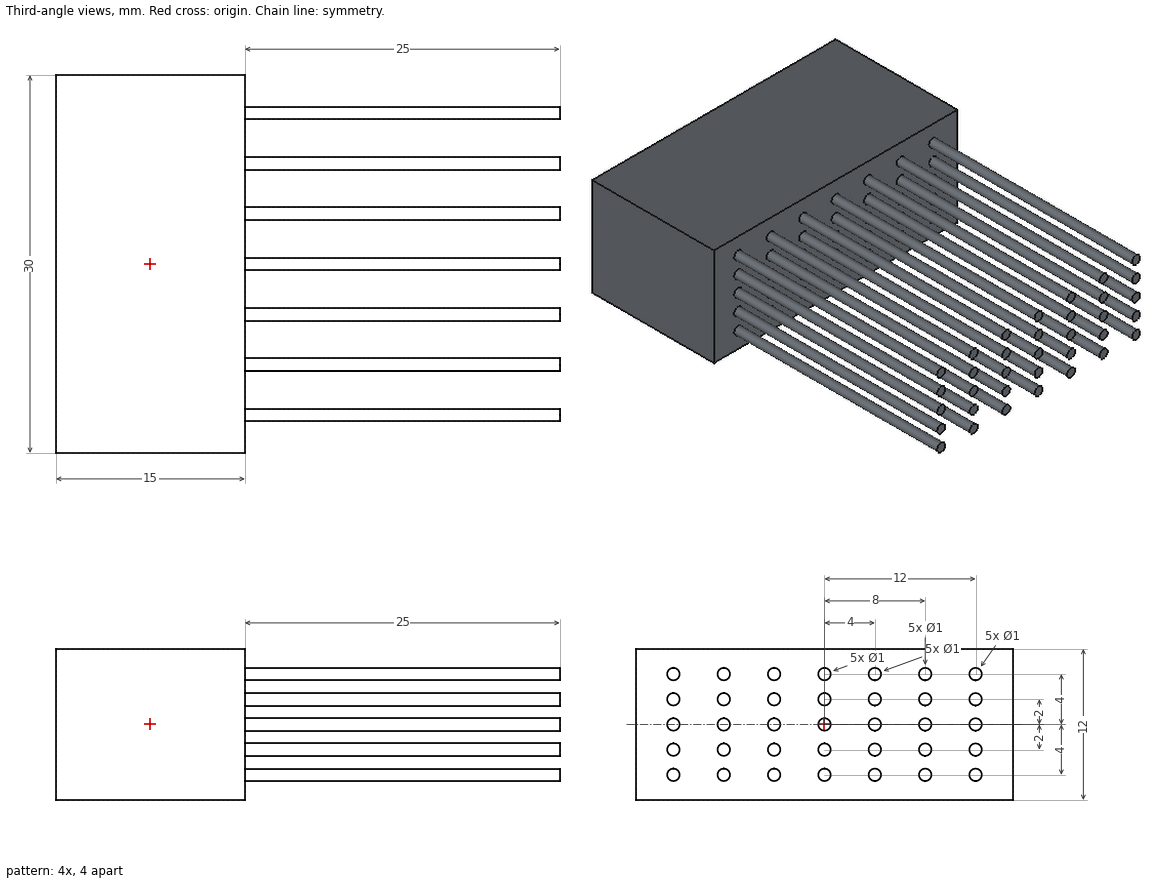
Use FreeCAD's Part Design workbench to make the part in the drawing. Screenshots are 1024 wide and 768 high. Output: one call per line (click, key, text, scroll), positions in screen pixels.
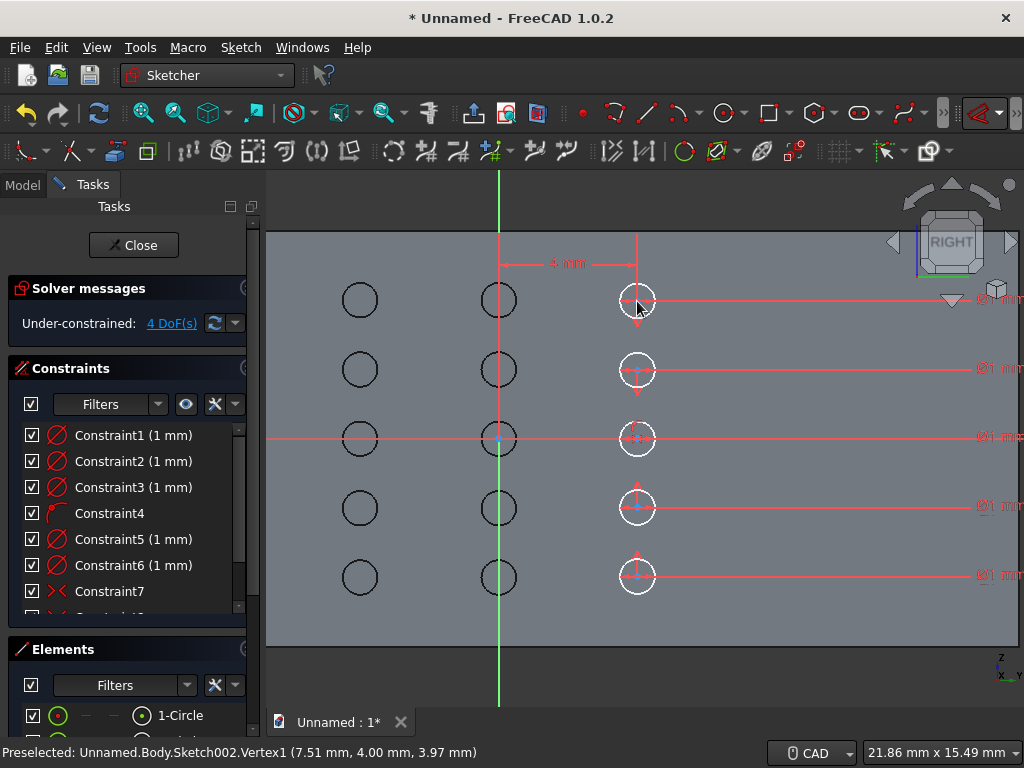
click(637, 301)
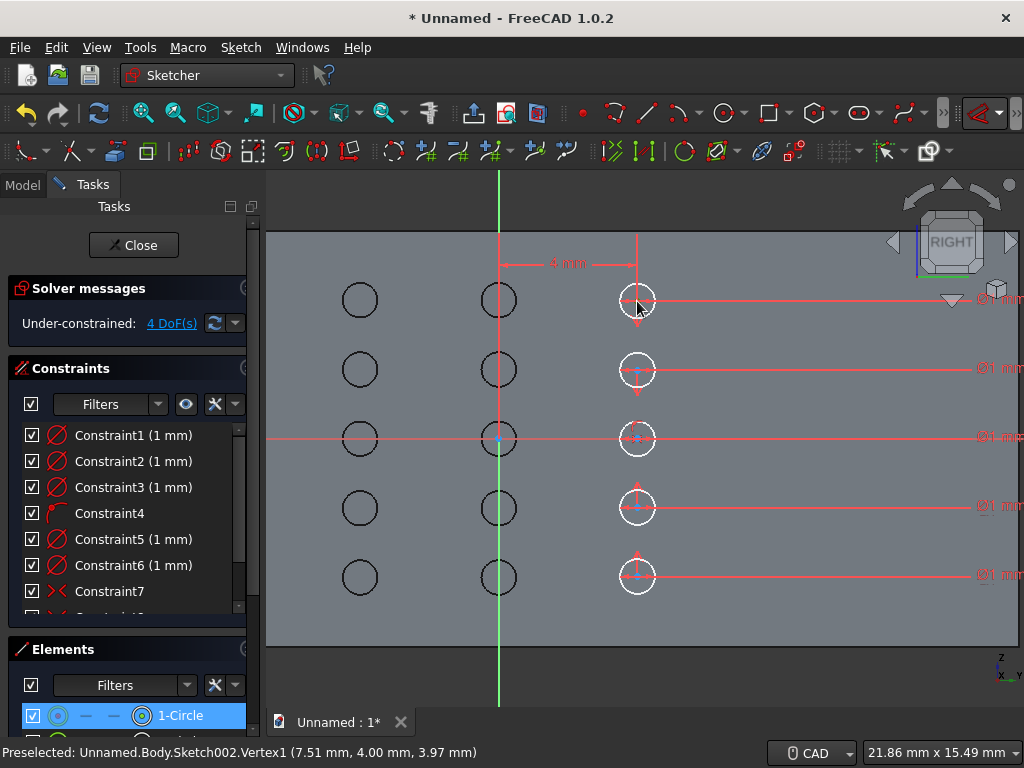
key(i)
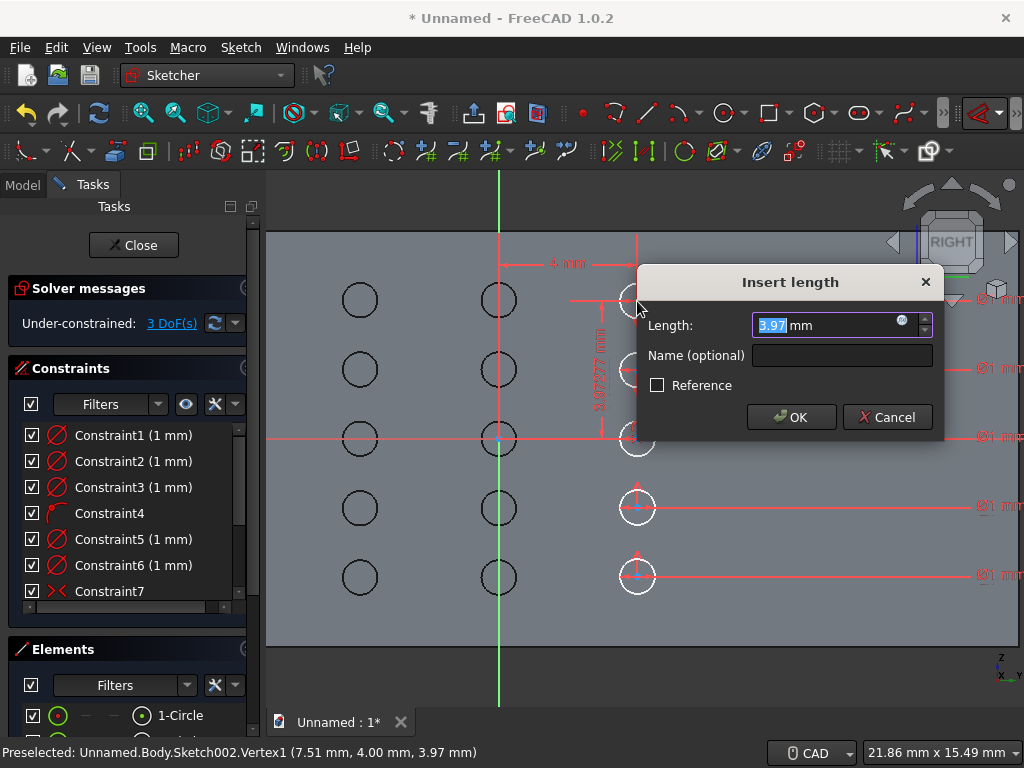
text(4)
key(Return)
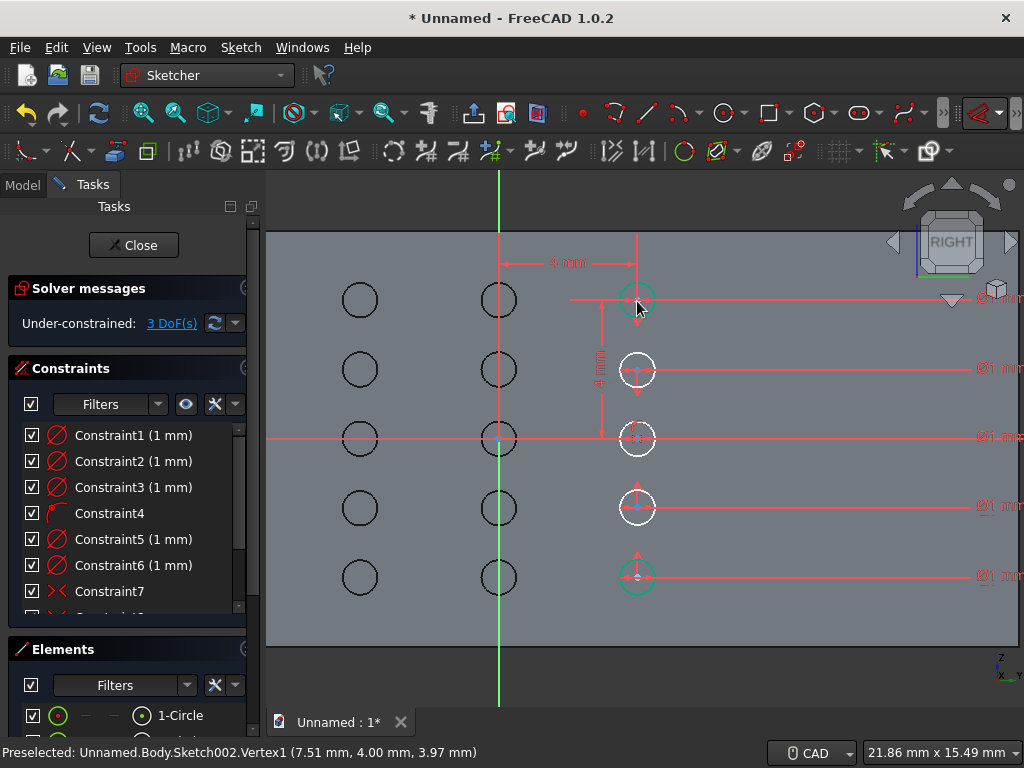
click(637, 370)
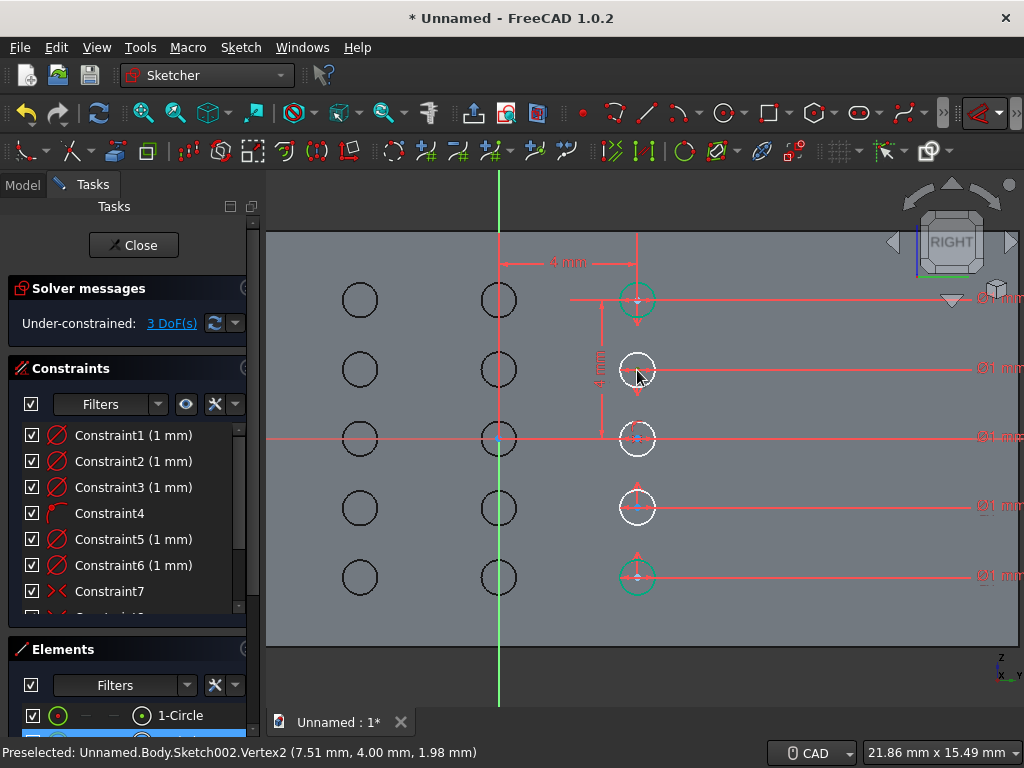
key(l)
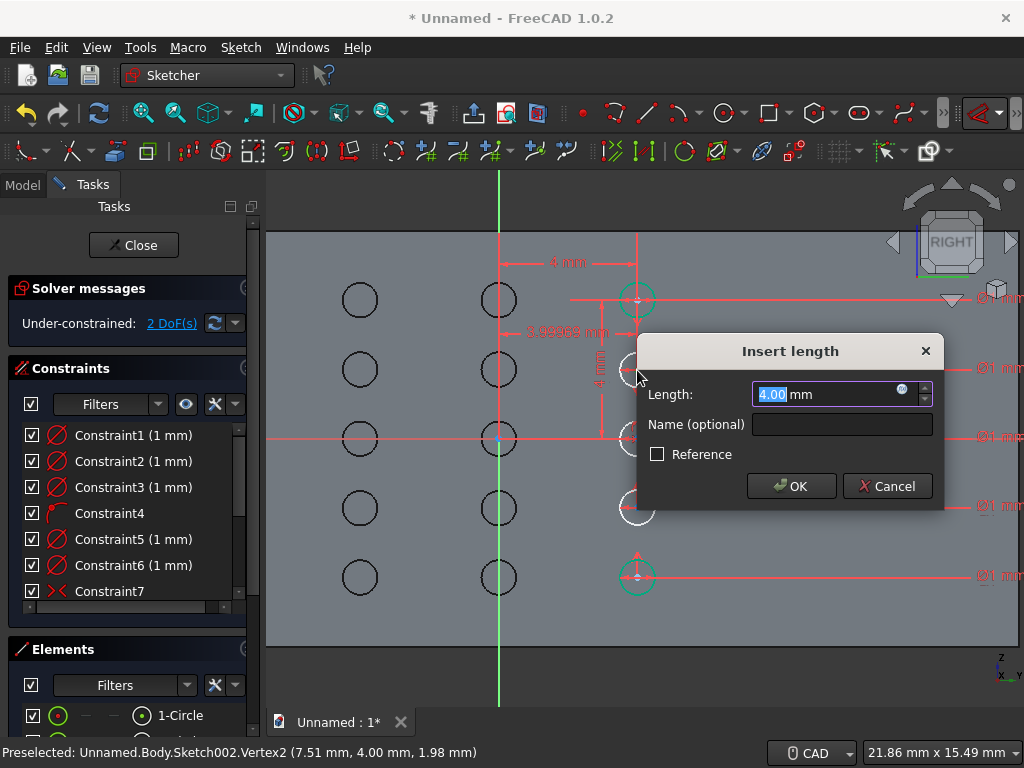
text(4)
key(Return)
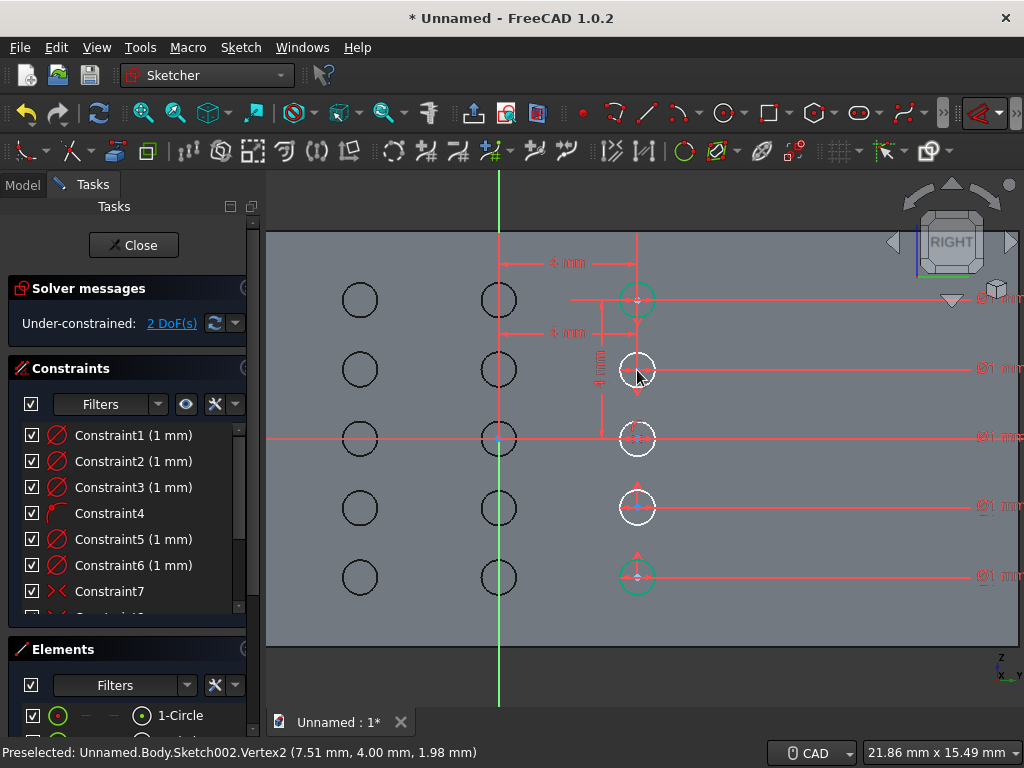
click(637, 370)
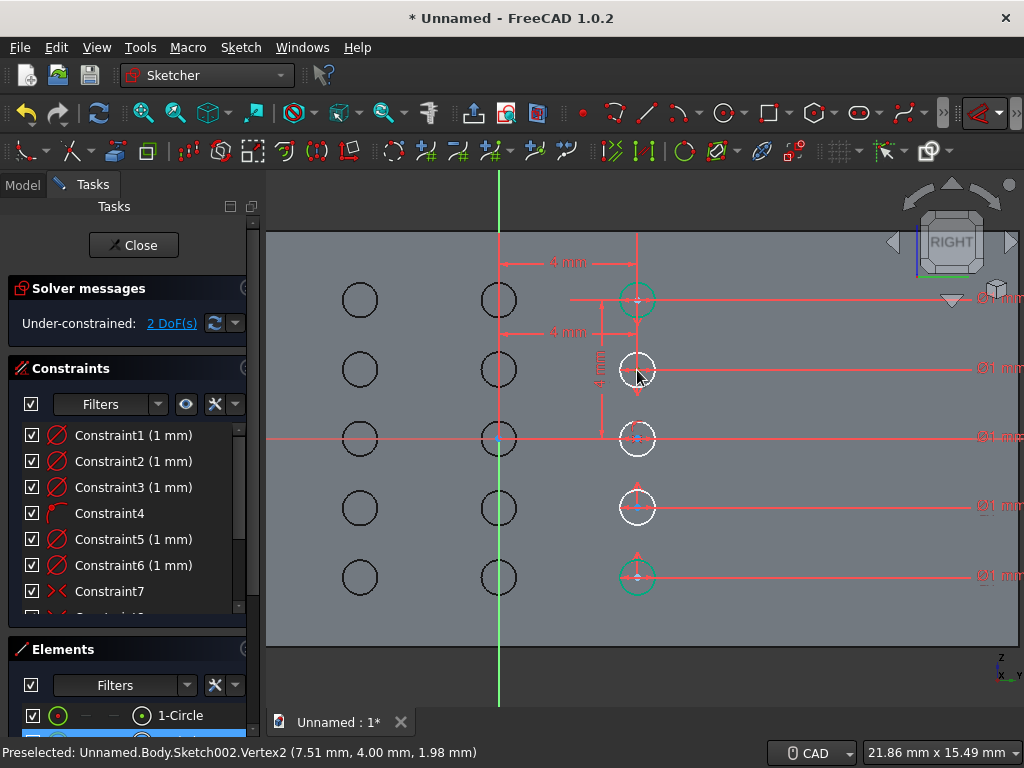
key(i)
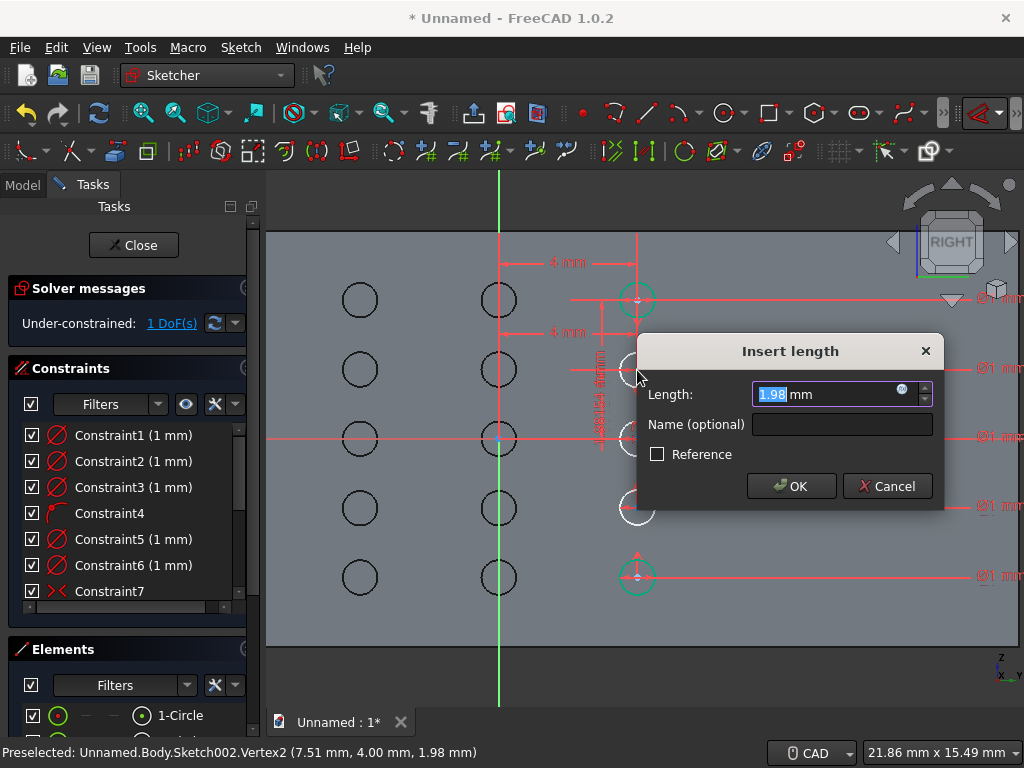
text(2)
key(Return)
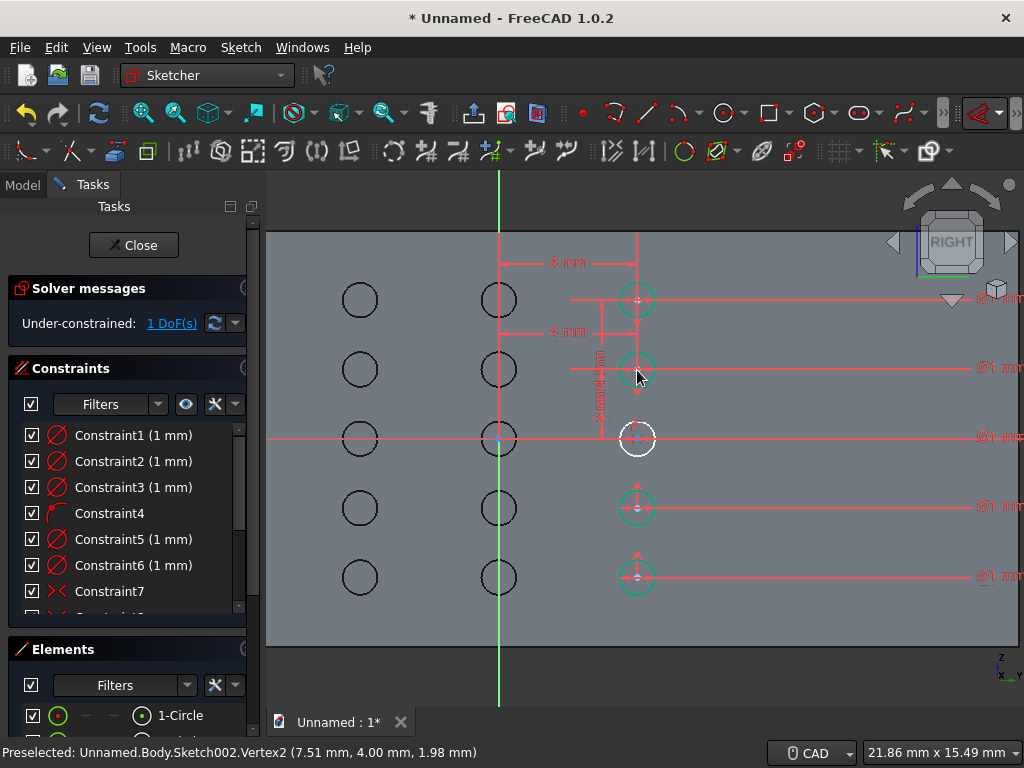
click(637, 439)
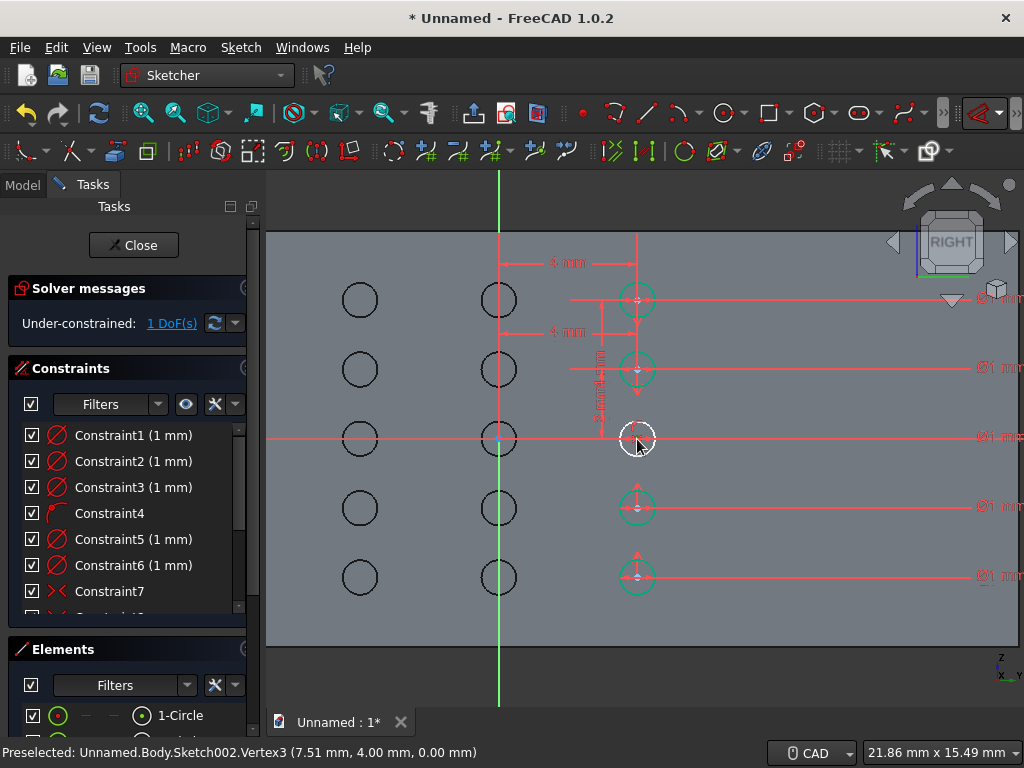
key(l)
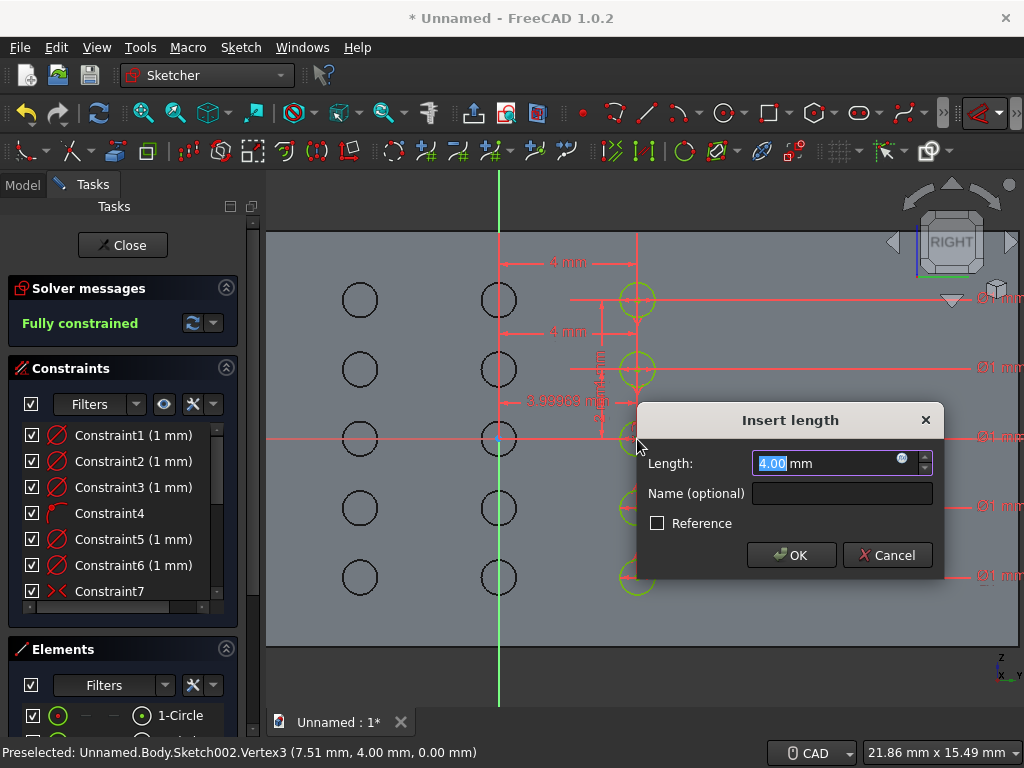
text(4)
key(Return)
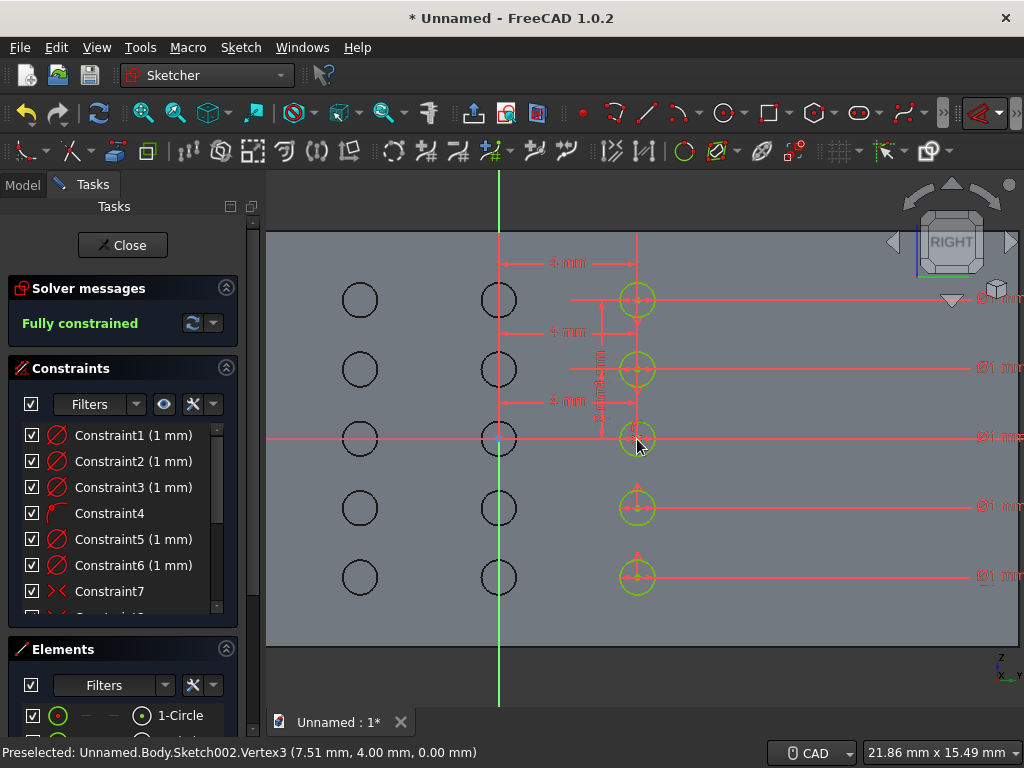
click(123, 245)